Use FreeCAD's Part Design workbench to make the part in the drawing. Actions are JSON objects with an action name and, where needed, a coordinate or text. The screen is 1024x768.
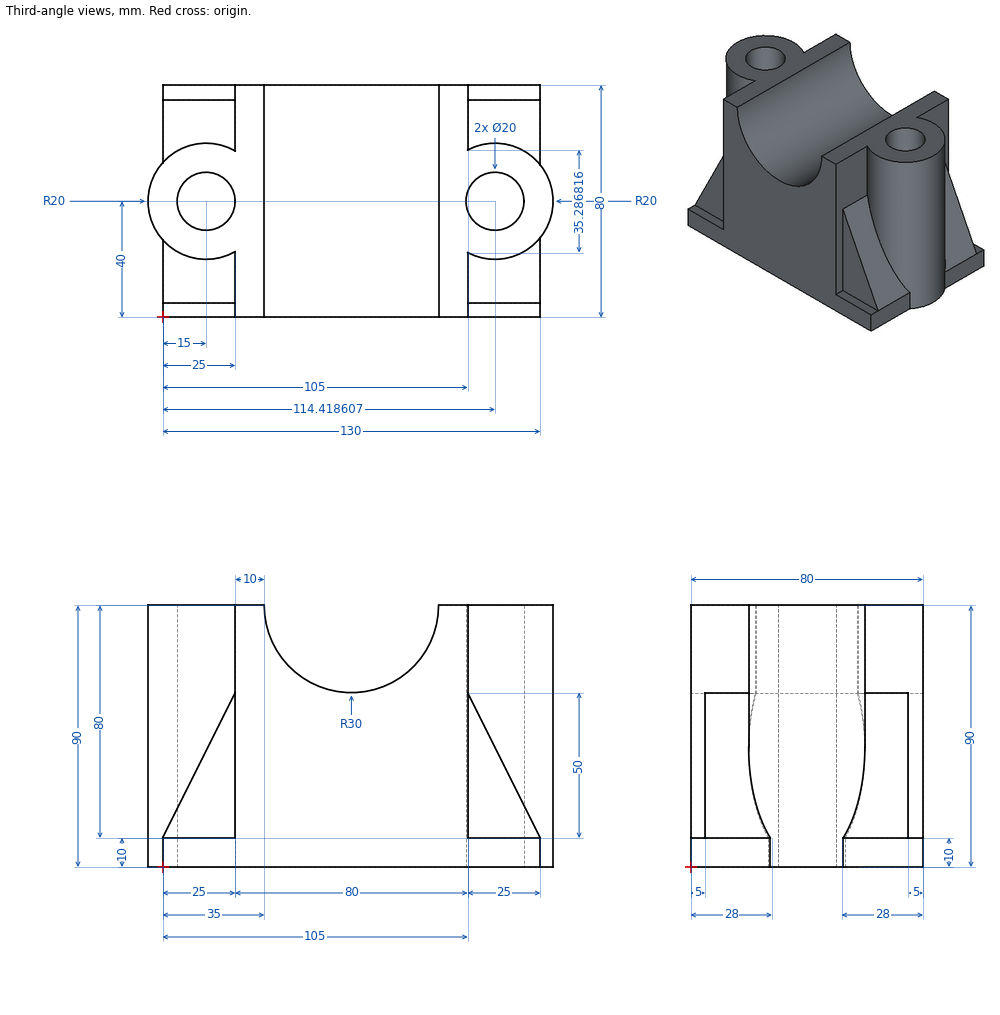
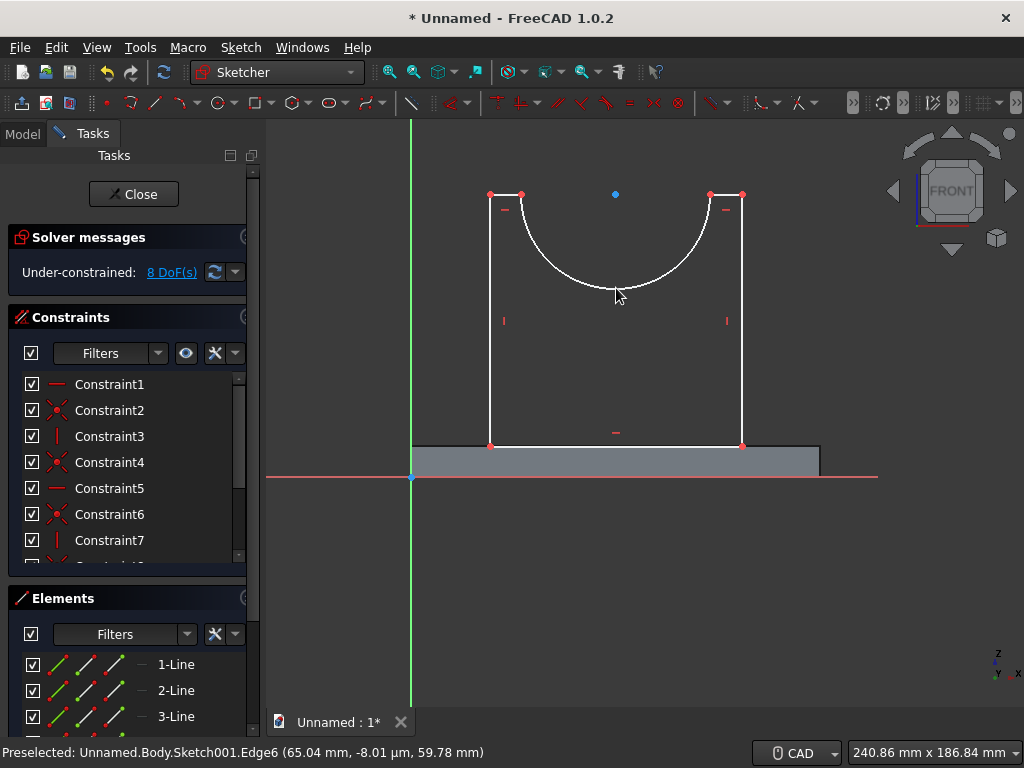
{"action": "left_click", "coordinate": [450, 104]}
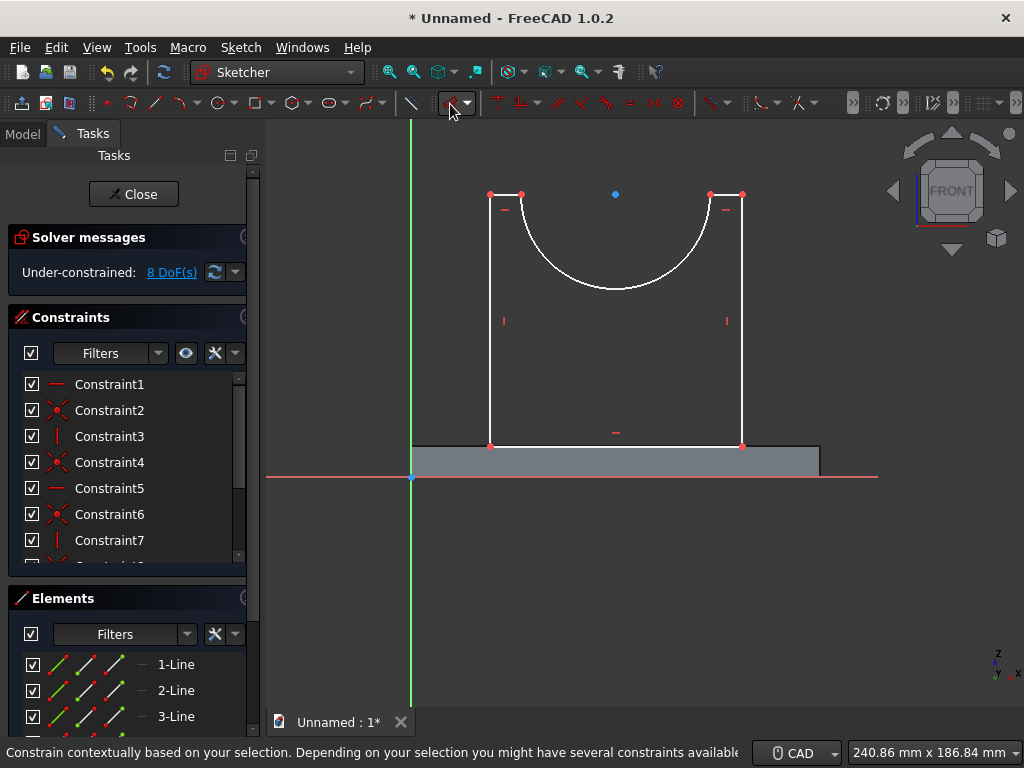
{"action": "left_click", "coordinate": [560, 271]}
{"action": "left_click", "coordinate": [541, 297]}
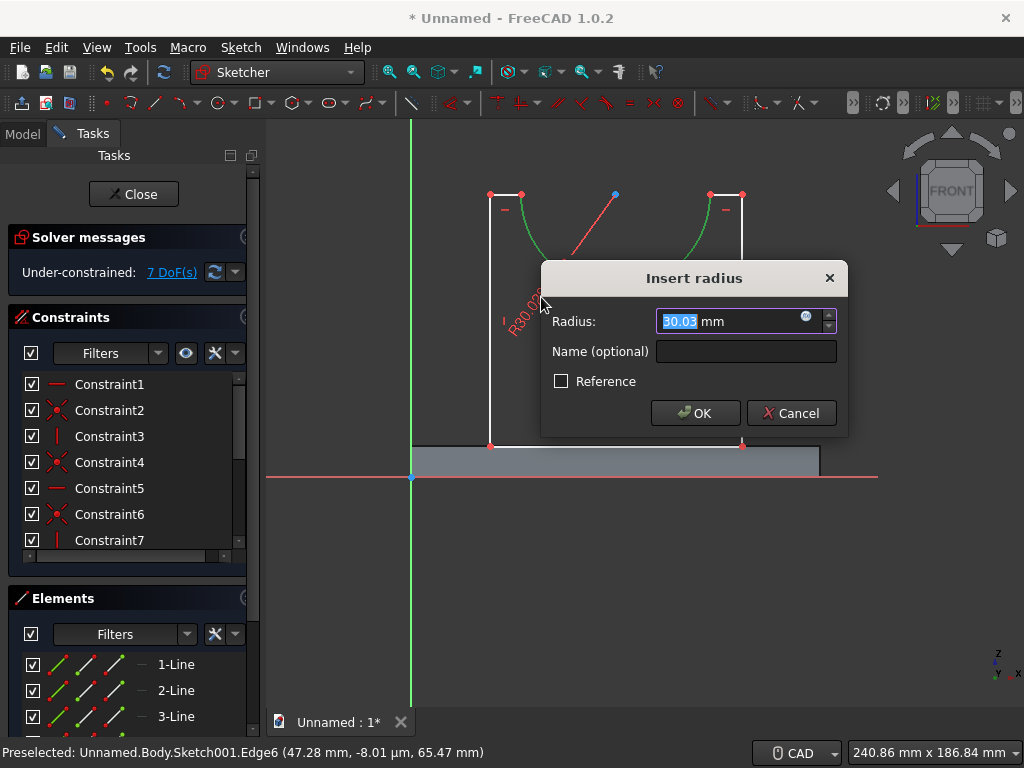
{"action": "type", "text": "30"}
{"action": "key", "text": "Return"}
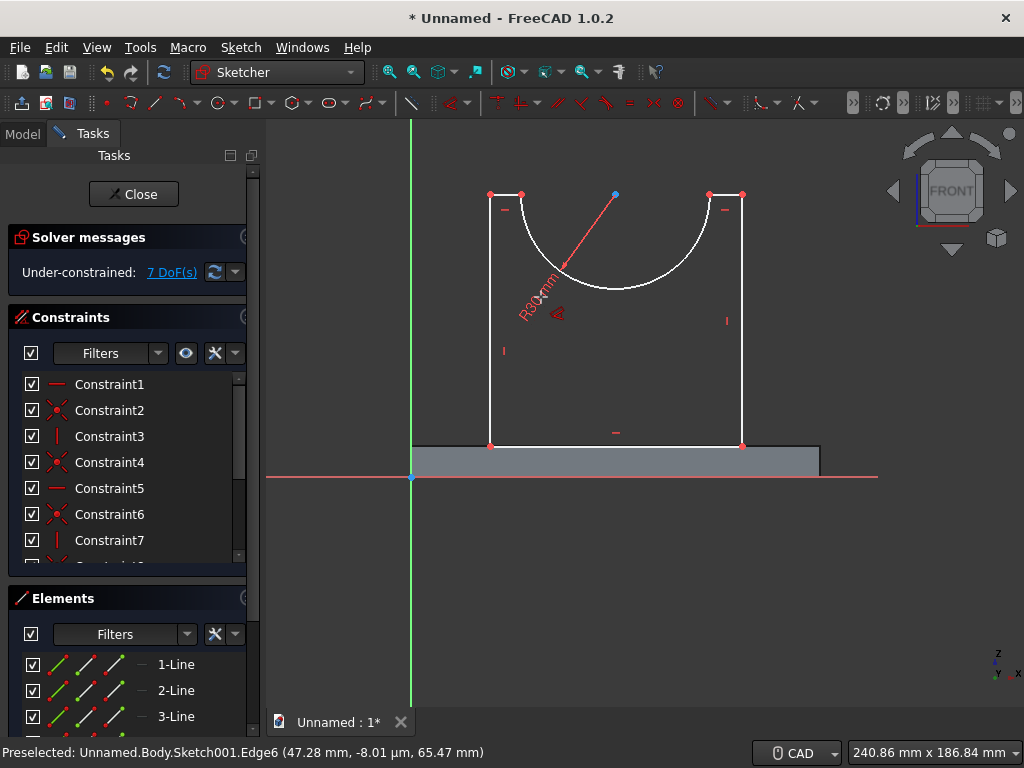
{"action": "scroll", "coordinate": [512, 195], "scroll_direction": "up", "scroll_amount": 2}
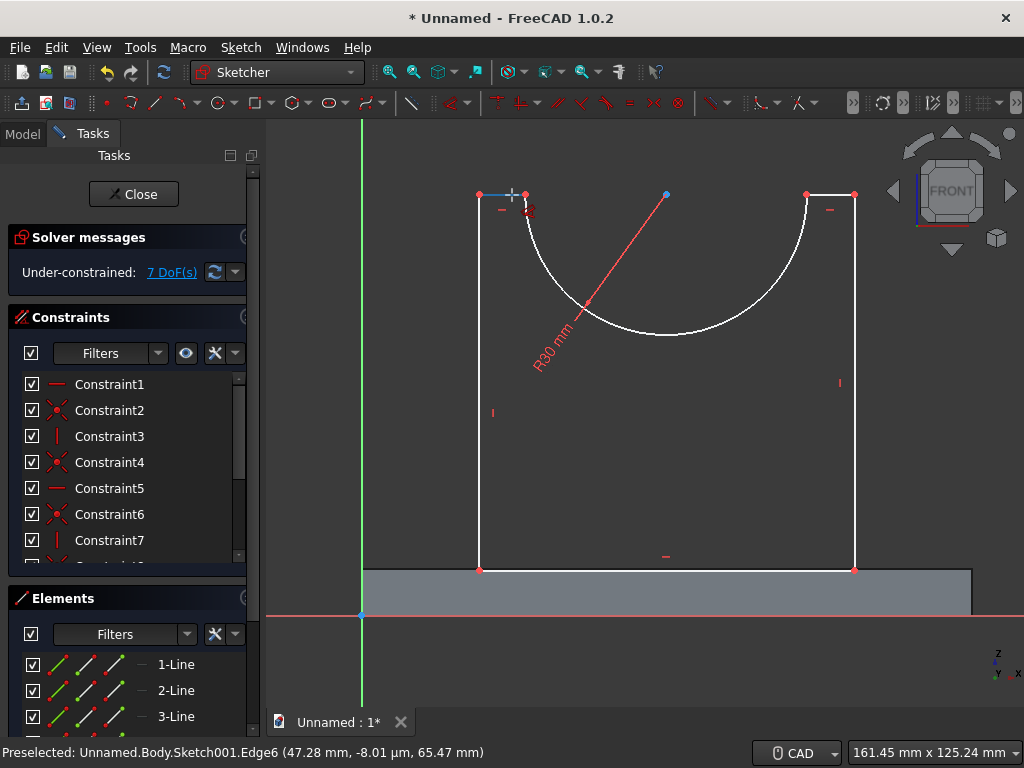
{"action": "left_click", "coordinate": [511, 195]}
{"action": "left_click", "coordinate": [502, 161]}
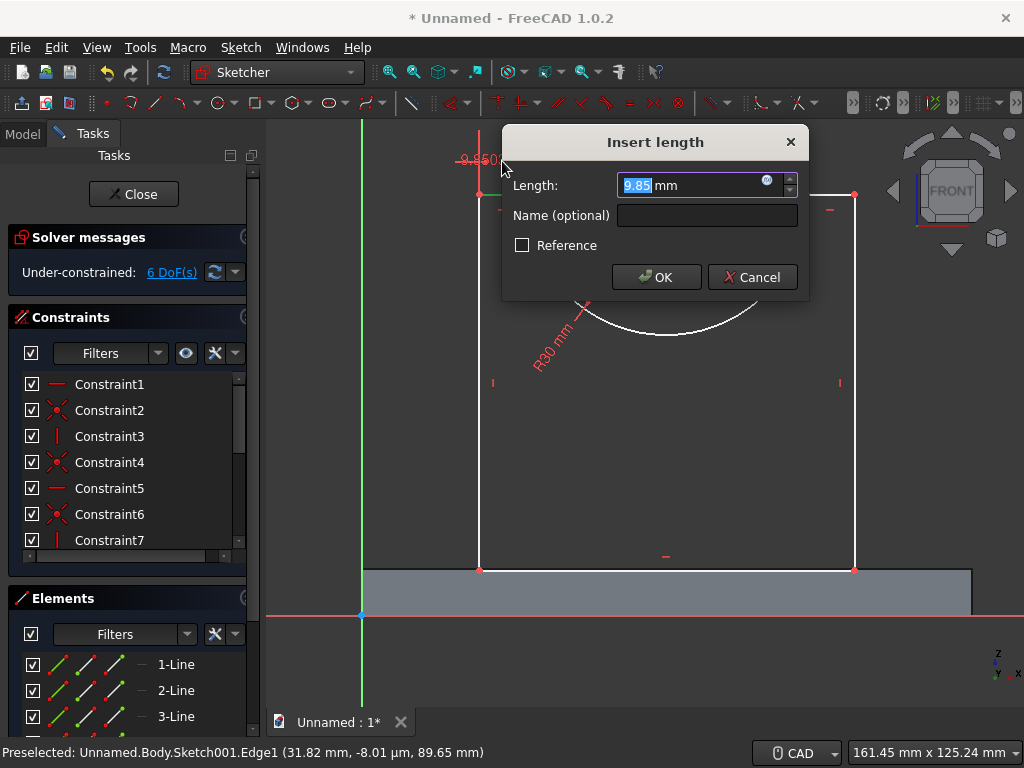
{"action": "type", "text": "10"}
{"action": "key", "text": "Return"}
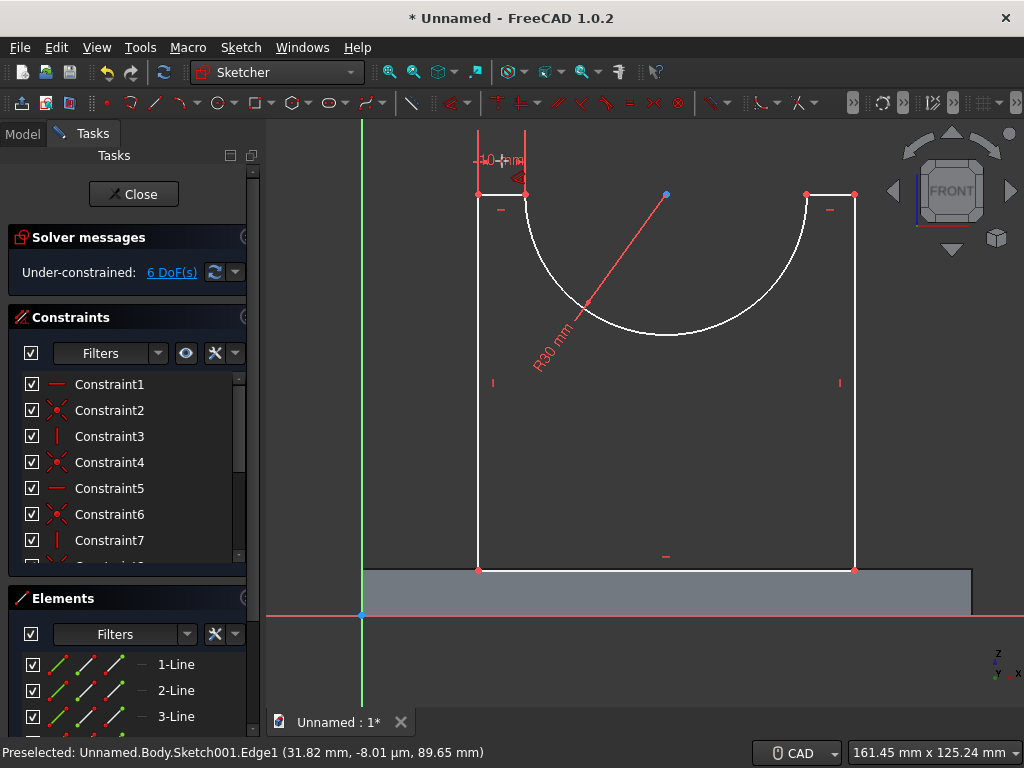
{"action": "left_click", "coordinate": [478, 308]}
{"action": "left_click", "coordinate": [444, 383]}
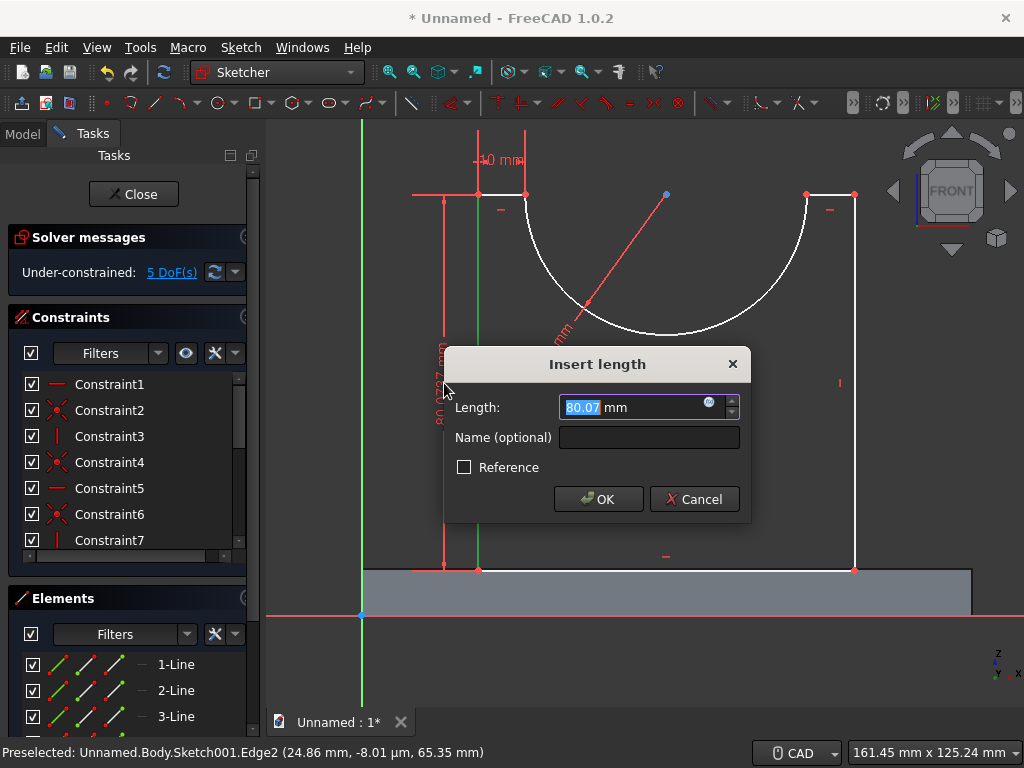
{"action": "type", "text": "80"}
{"action": "key", "text": "Return"}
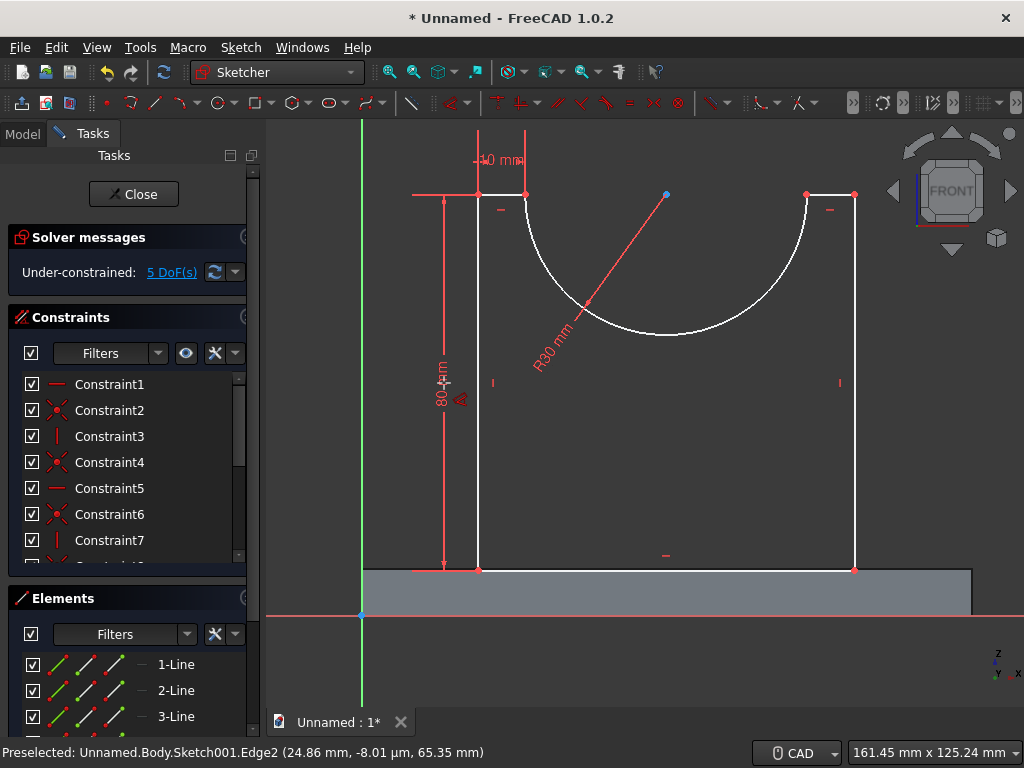
{"action": "left_click", "coordinate": [591, 571]}
{"action": "left_click", "coordinate": [667, 537]}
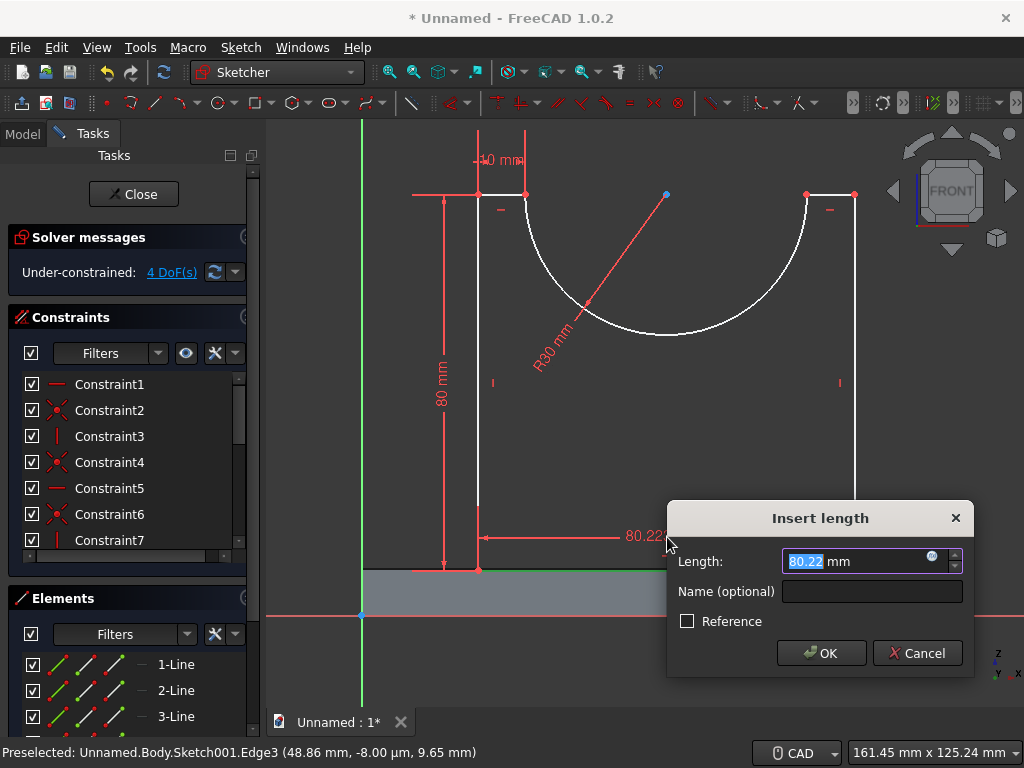
{"action": "type", "text": "80"}
{"action": "key", "text": "Return"}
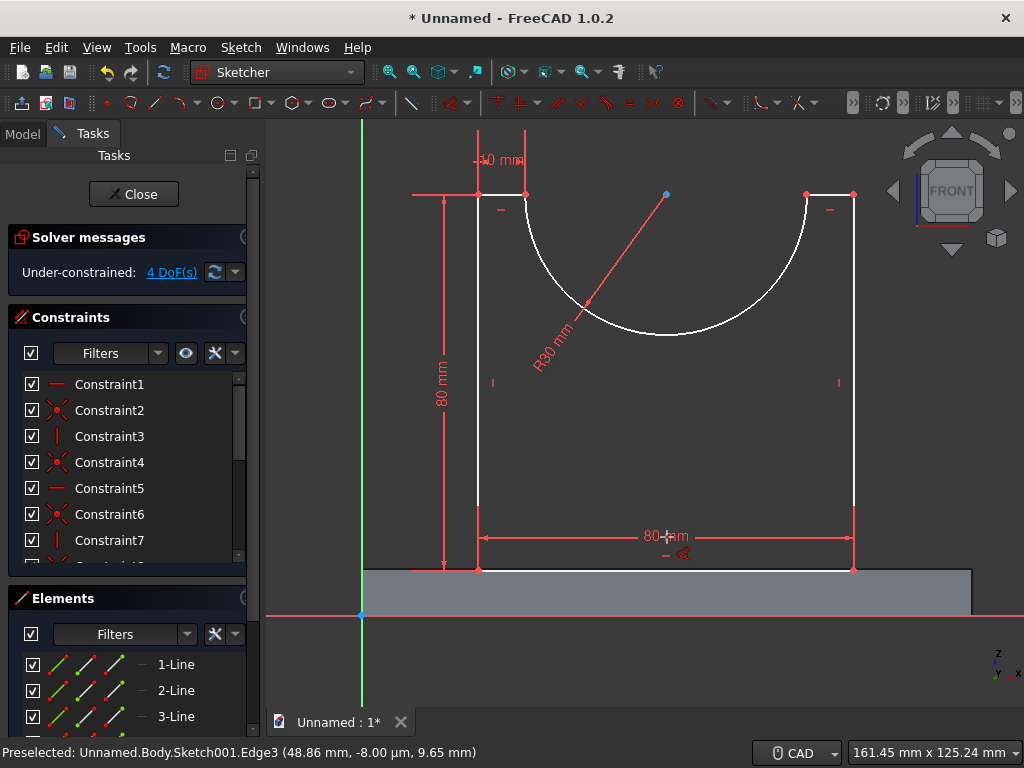
{"action": "left_click", "coordinate": [854, 458]}
{"action": "left_click", "coordinate": [820, 383]}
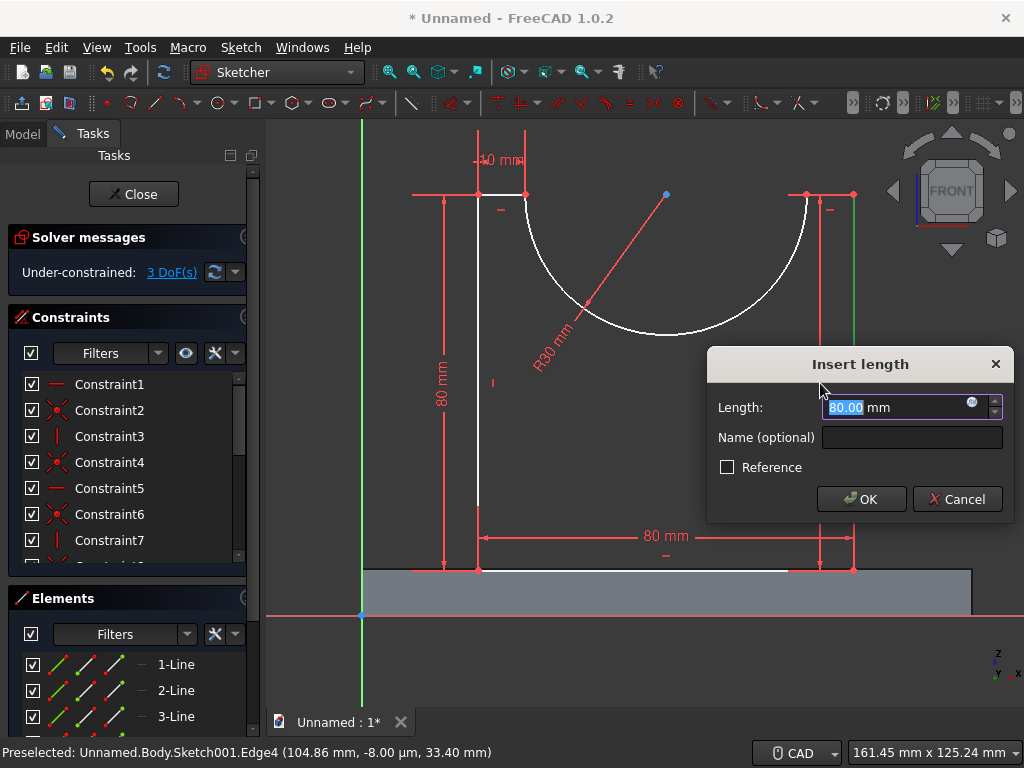
{"action": "type", "text": "80"}
{"action": "key", "text": "Return"}